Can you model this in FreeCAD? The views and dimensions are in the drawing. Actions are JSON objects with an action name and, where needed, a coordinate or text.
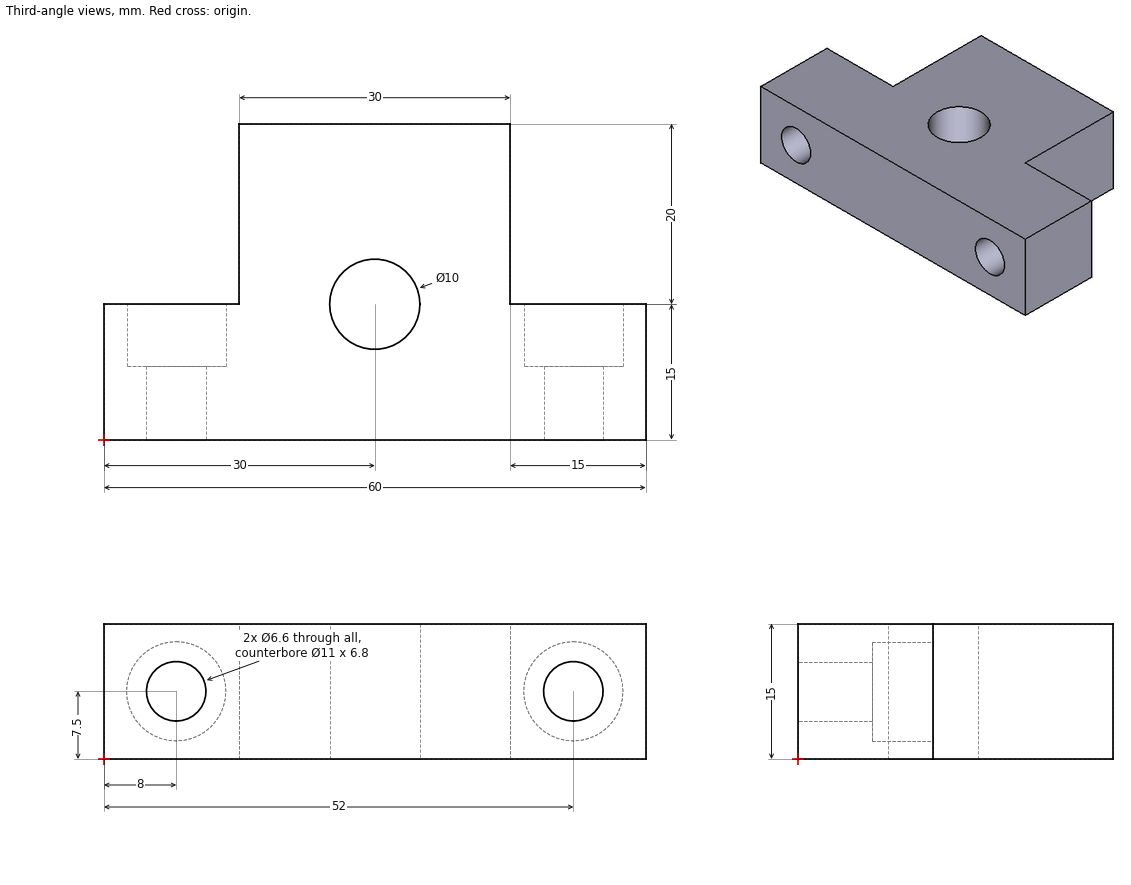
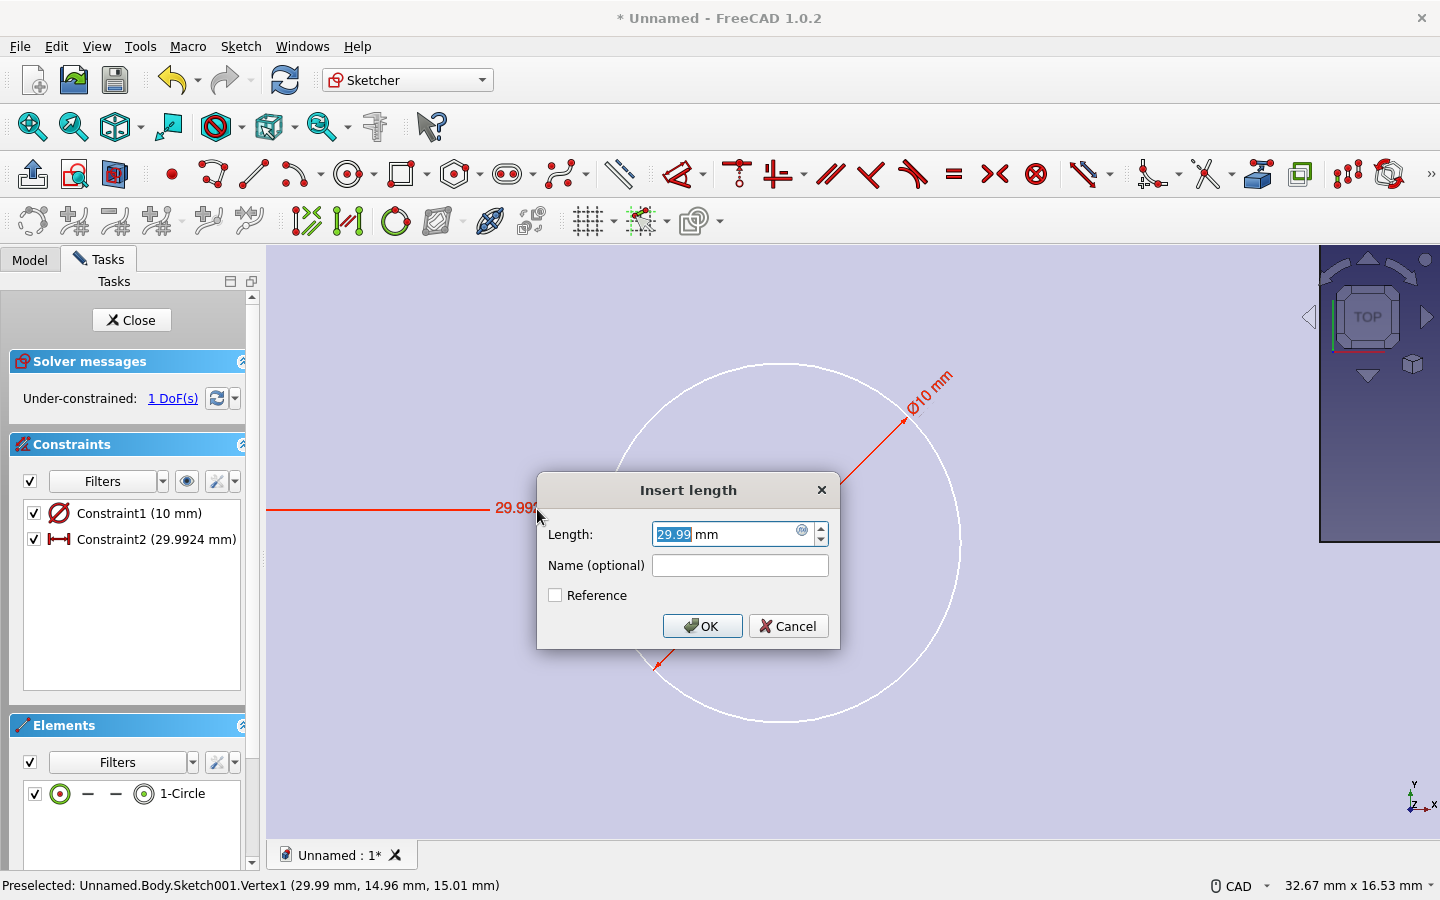
{"action": "type", "text": "30"}
{"action": "key", "text": "Return"}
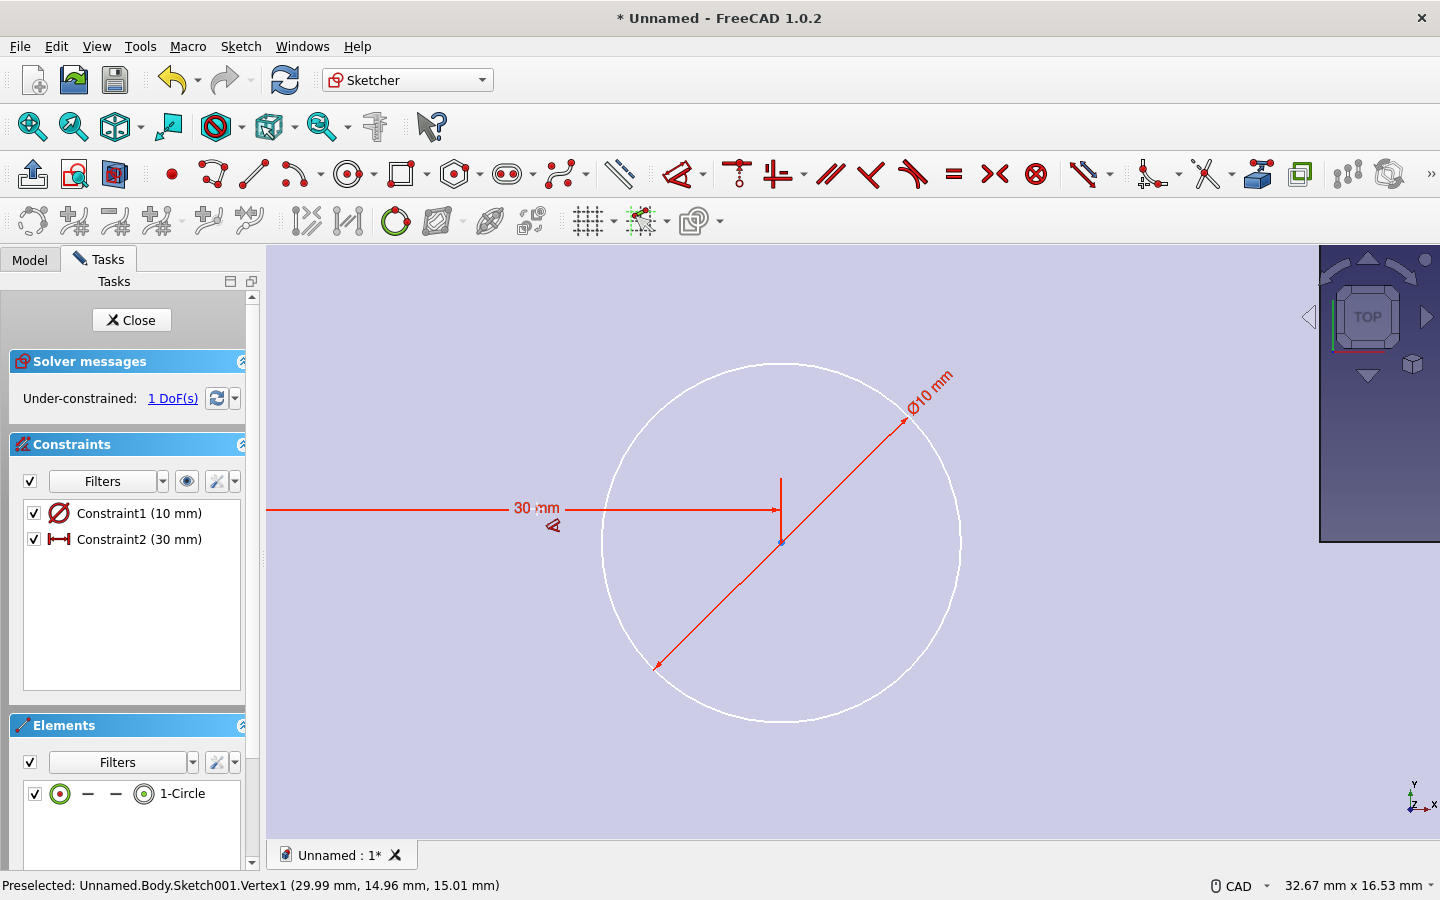
{"action": "left_click", "coordinate": [781, 543]}
{"action": "left_click", "coordinate": [815, 677]}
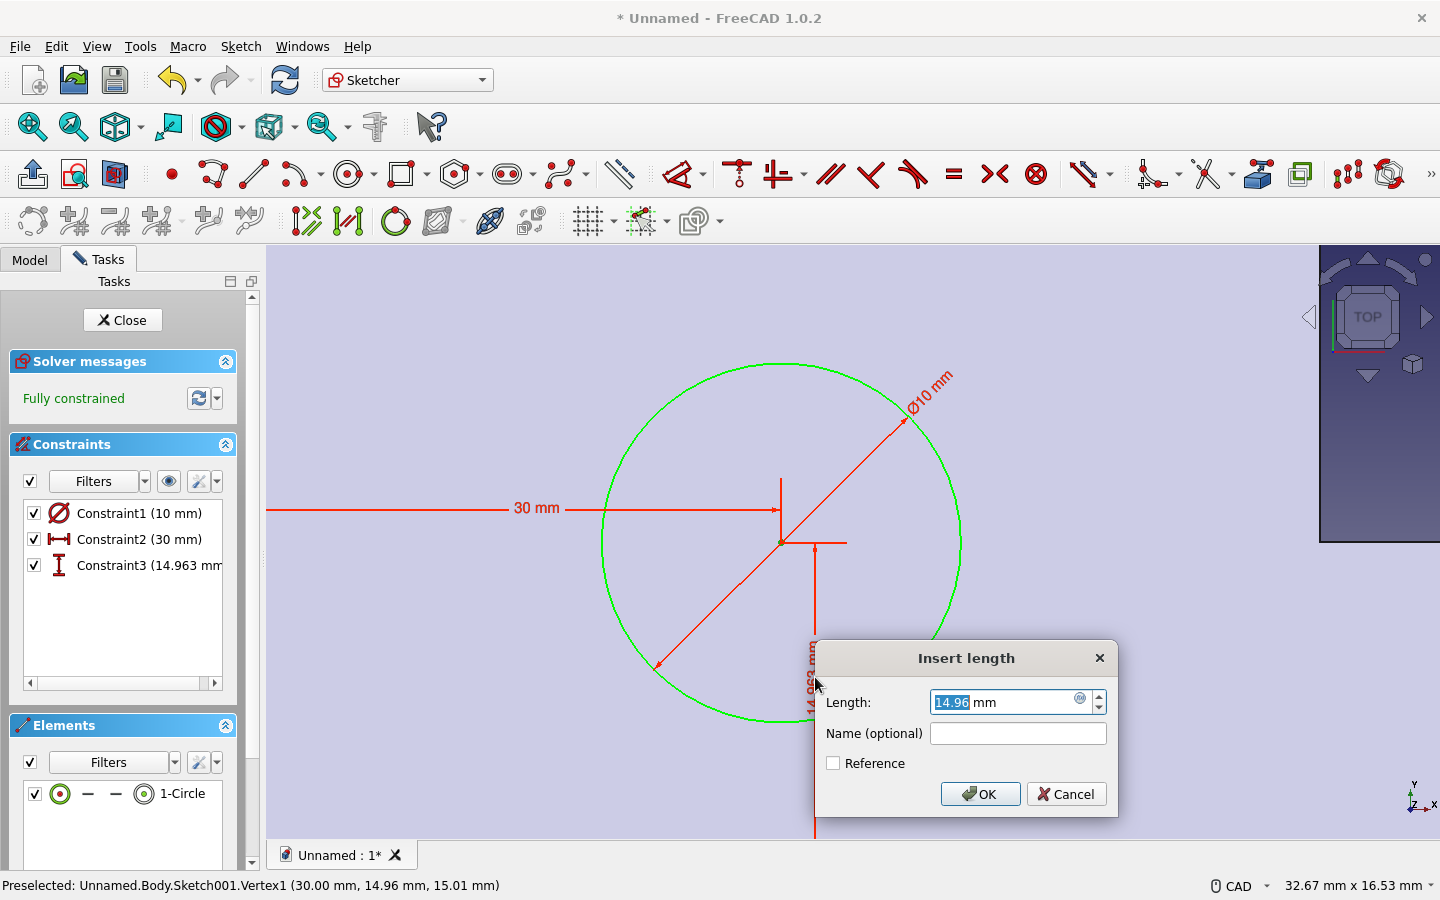
{"action": "type", "text": "15"}
{"action": "key", "text": "Return"}
{"action": "key", "text": "Escape"}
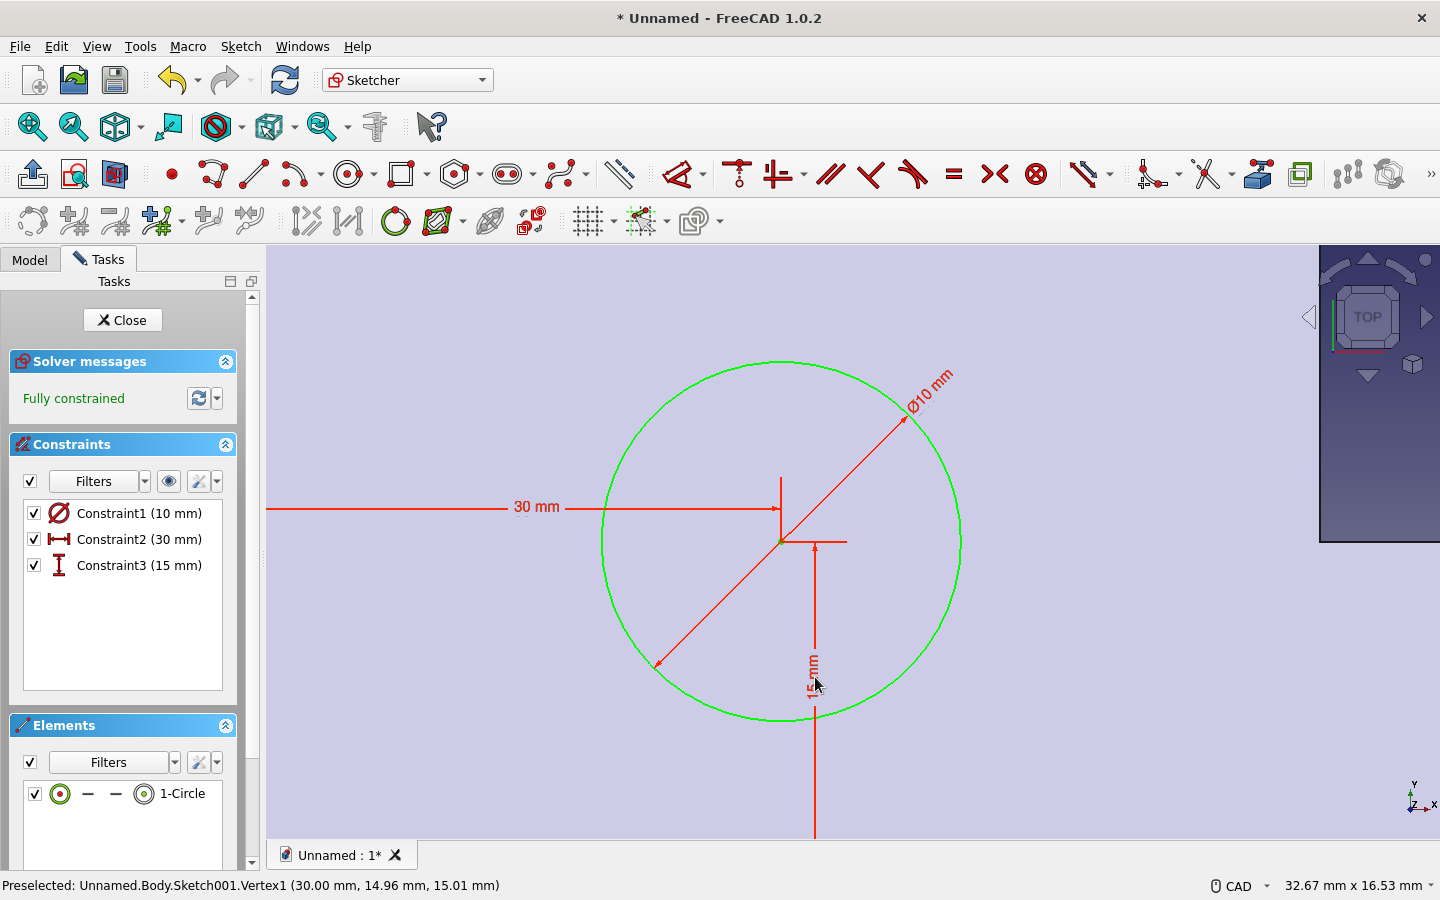
{"action": "left_click", "coordinate": [123, 320]}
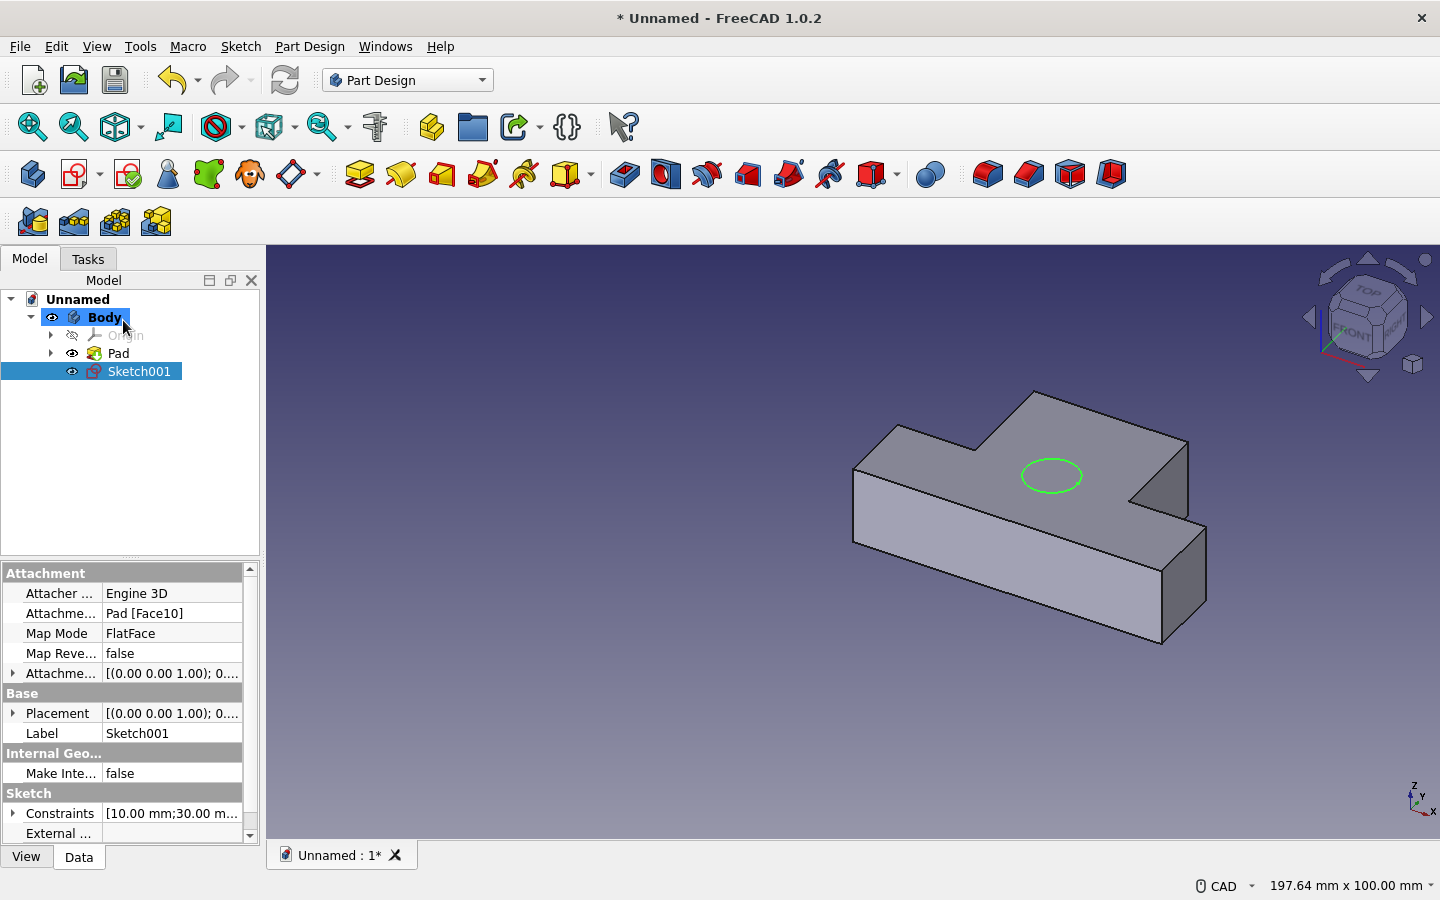
{"action": "left_click", "coordinate": [625, 174]}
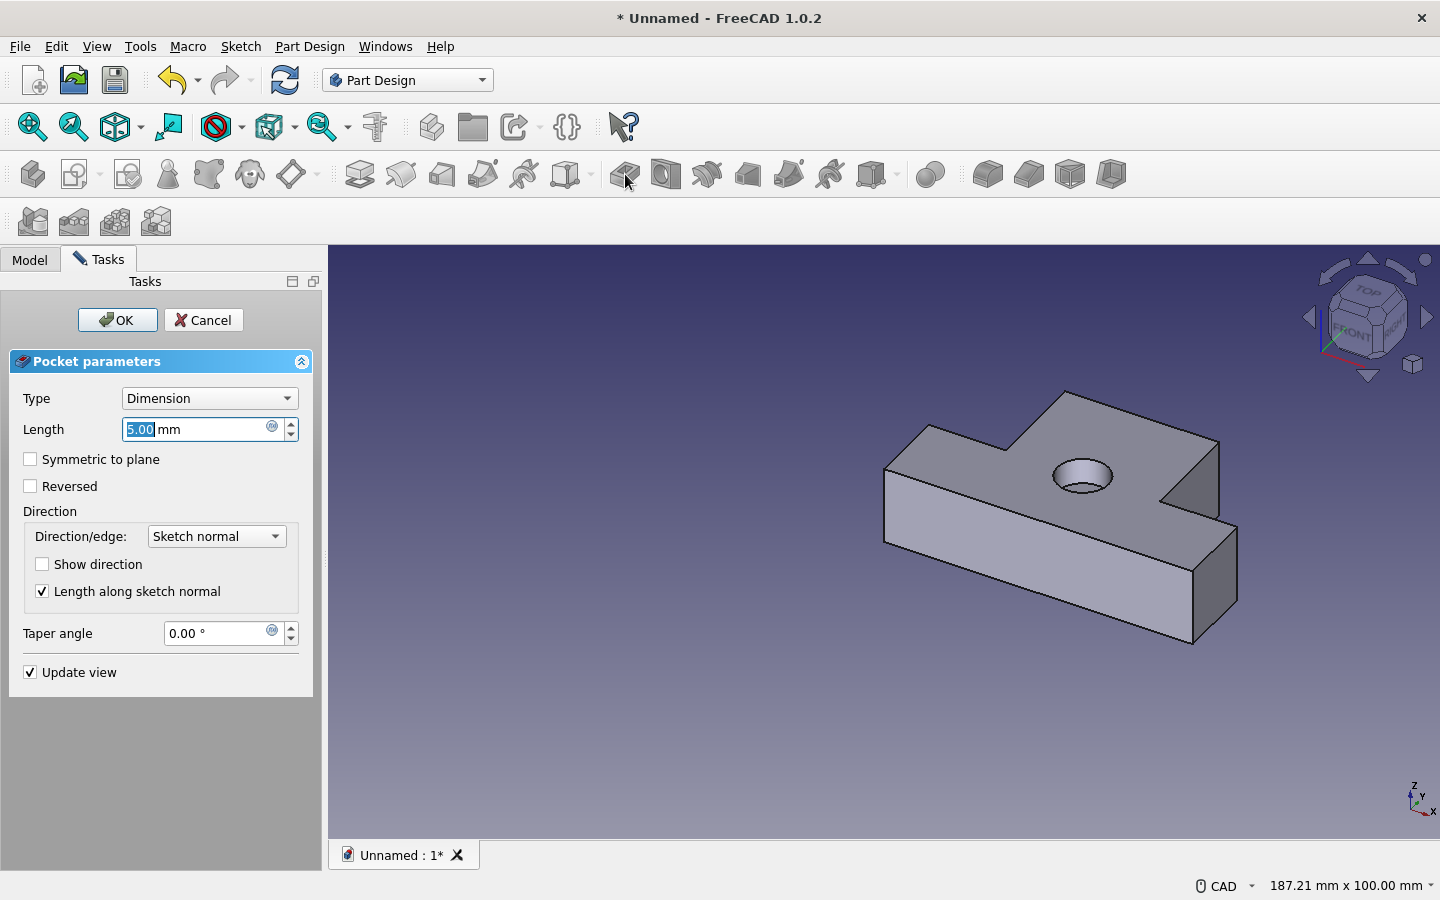
{"action": "left_click", "coordinate": [210, 398]}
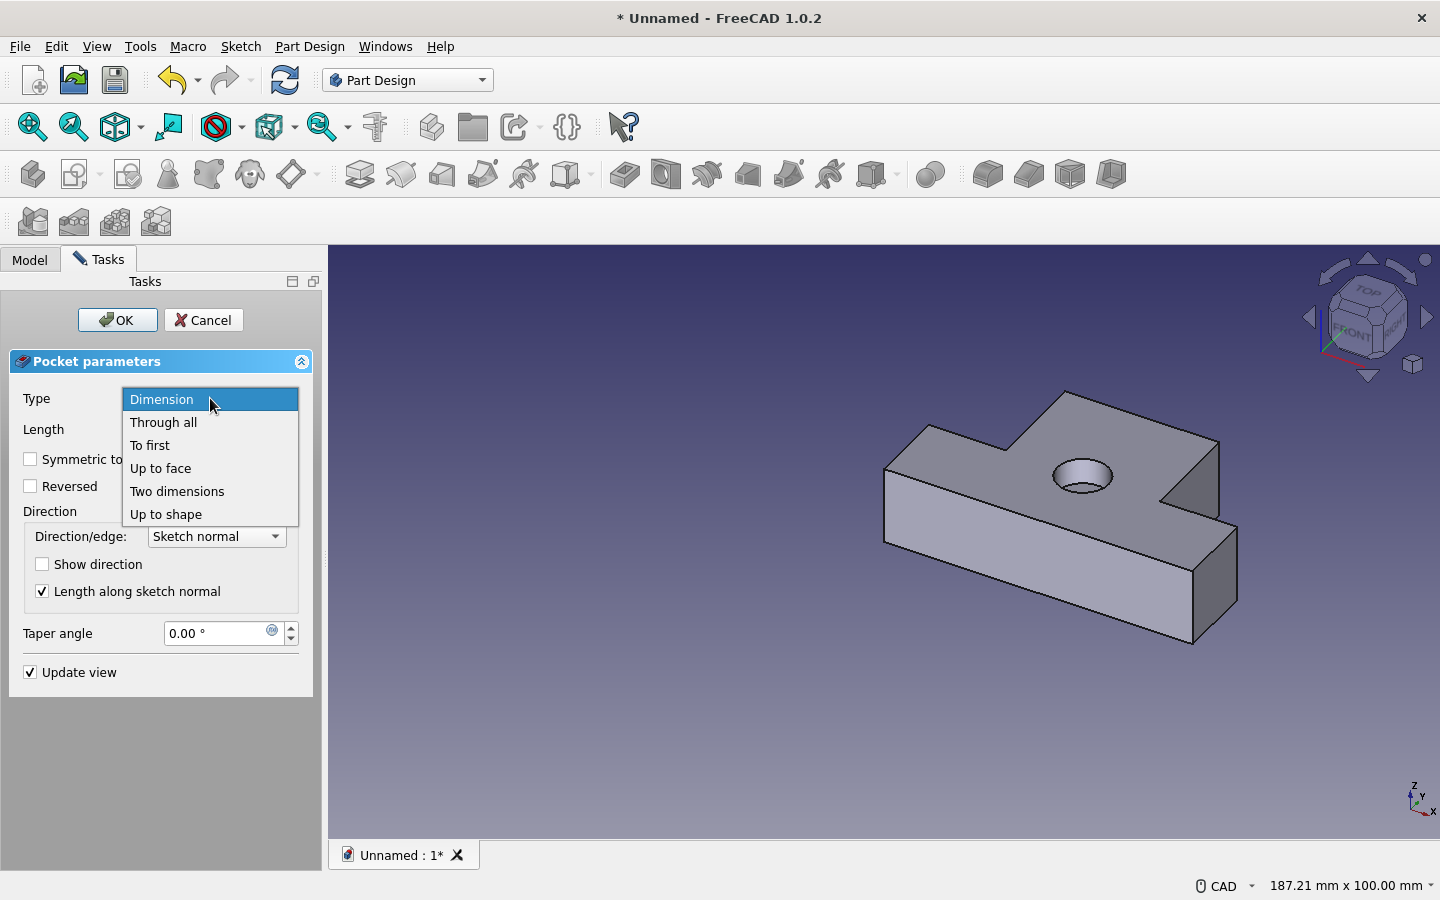
{"action": "left_click", "coordinate": [208, 422]}